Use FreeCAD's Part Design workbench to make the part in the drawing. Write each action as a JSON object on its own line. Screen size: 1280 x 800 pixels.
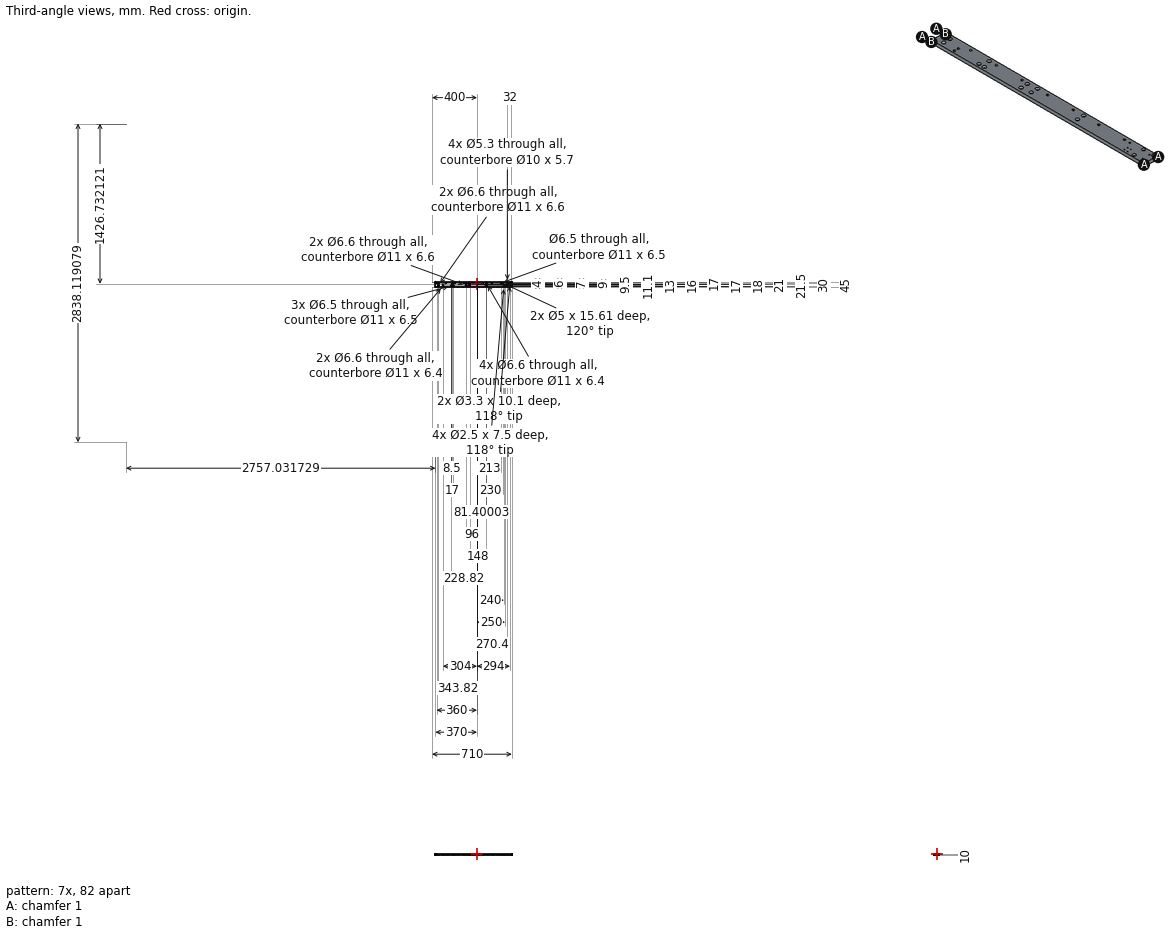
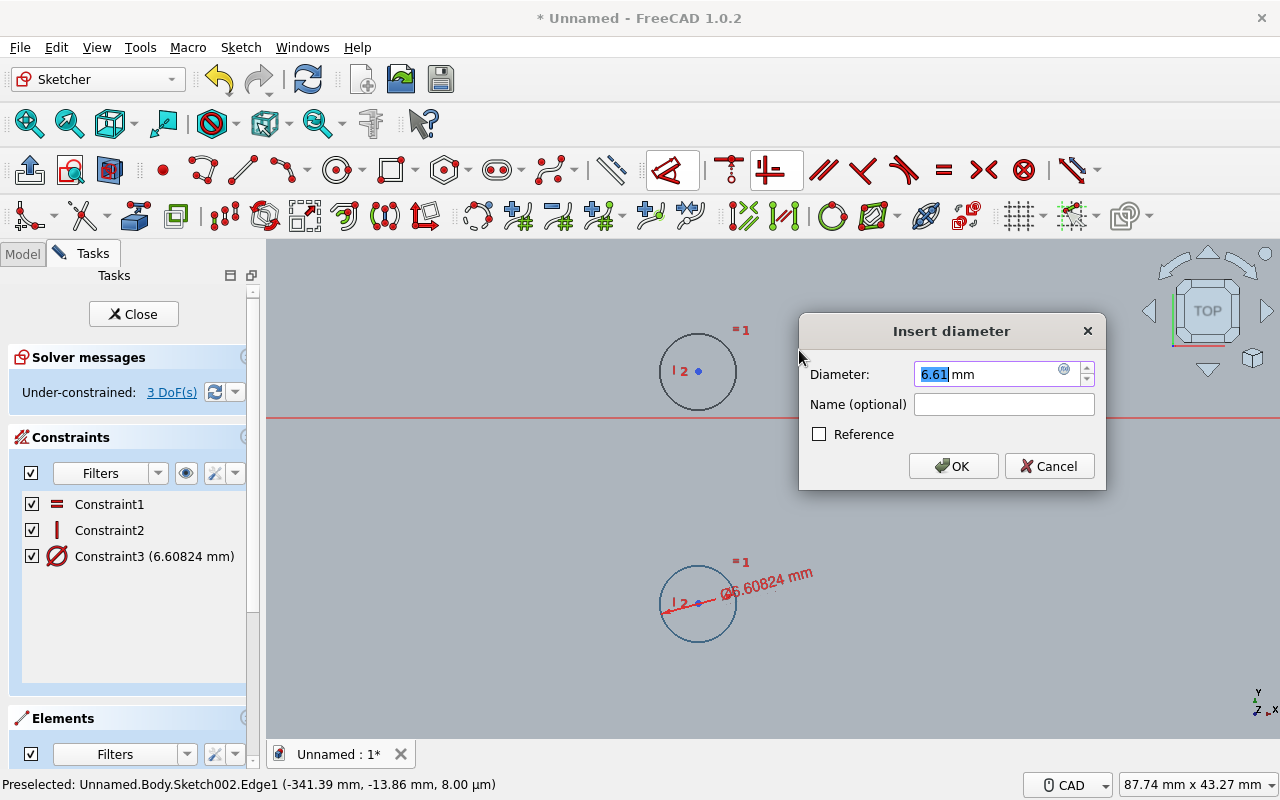
{"action": "type", "text": "6.6"}
{"action": "key", "text": "Return"}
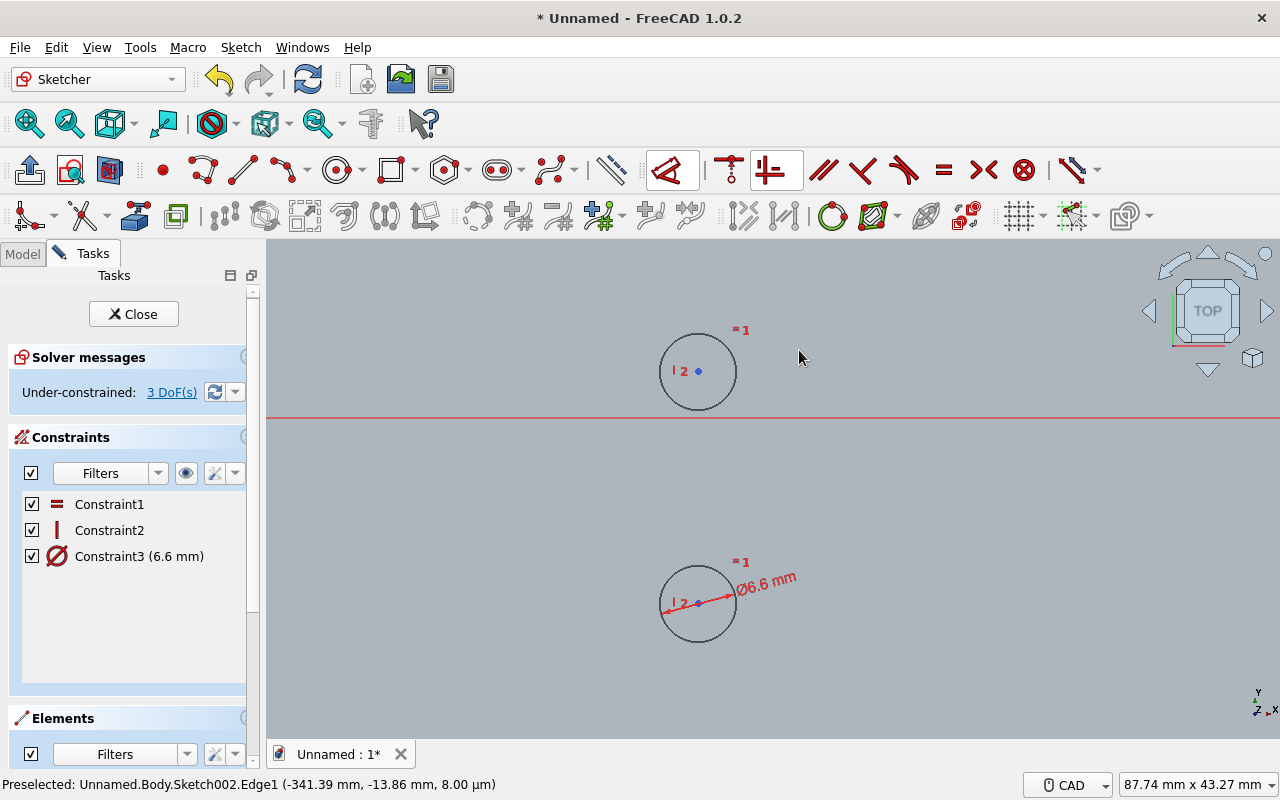
{"action": "left_click", "coordinate": [698, 372]}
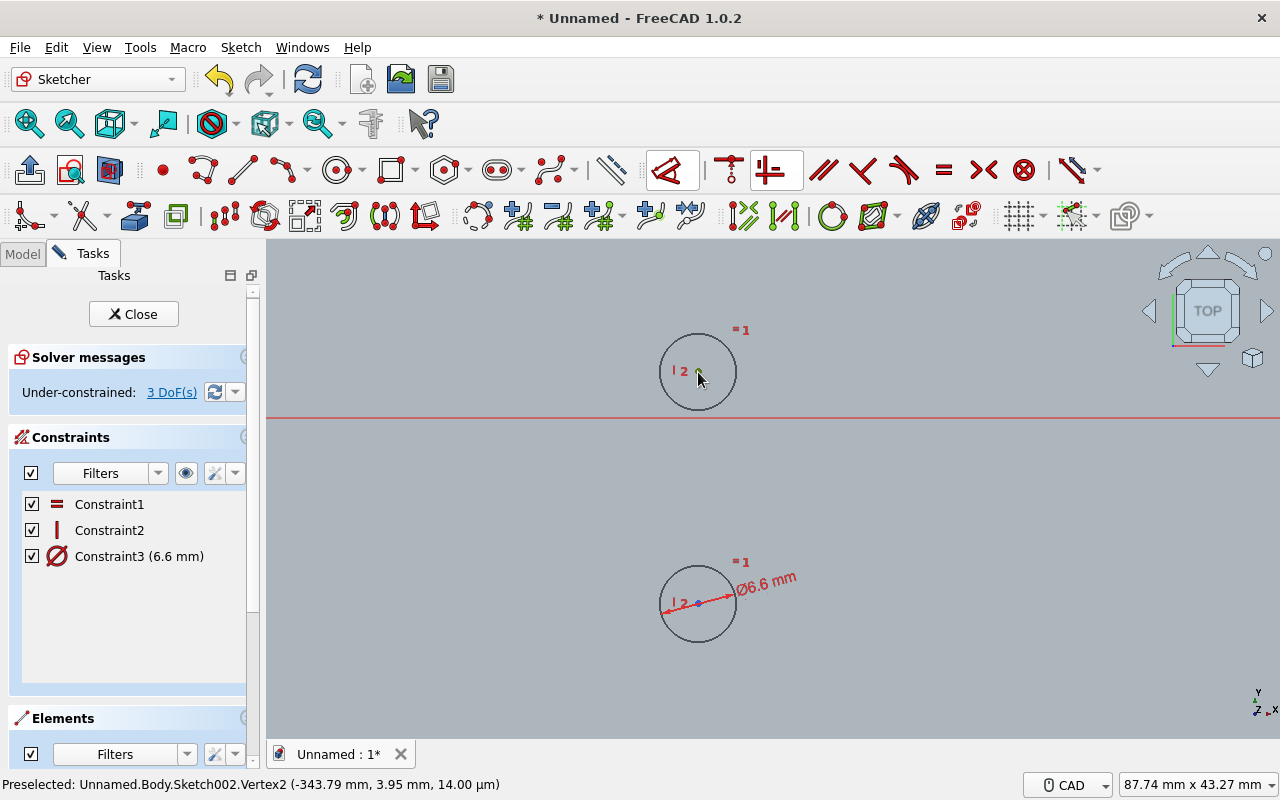
{"action": "left_click", "coordinate": [694, 170]}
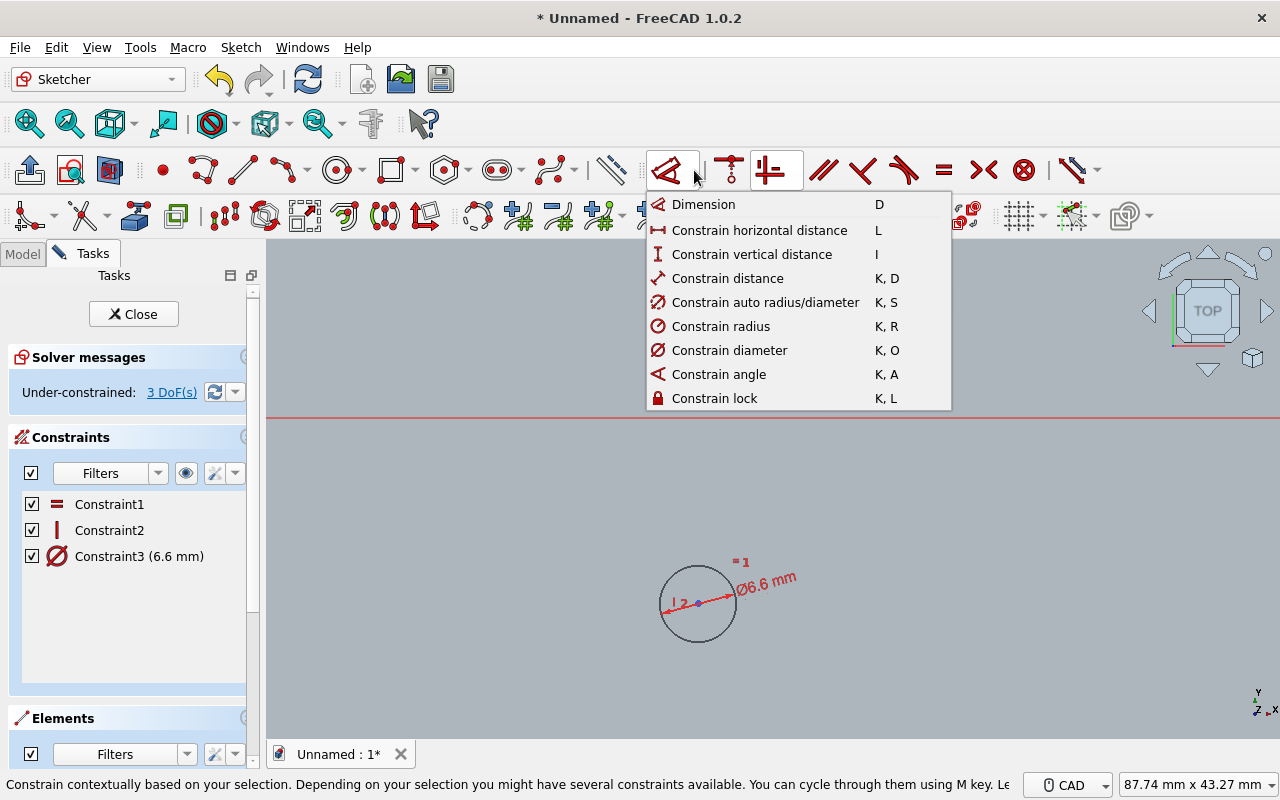
{"action": "left_click", "coordinate": [799, 254]}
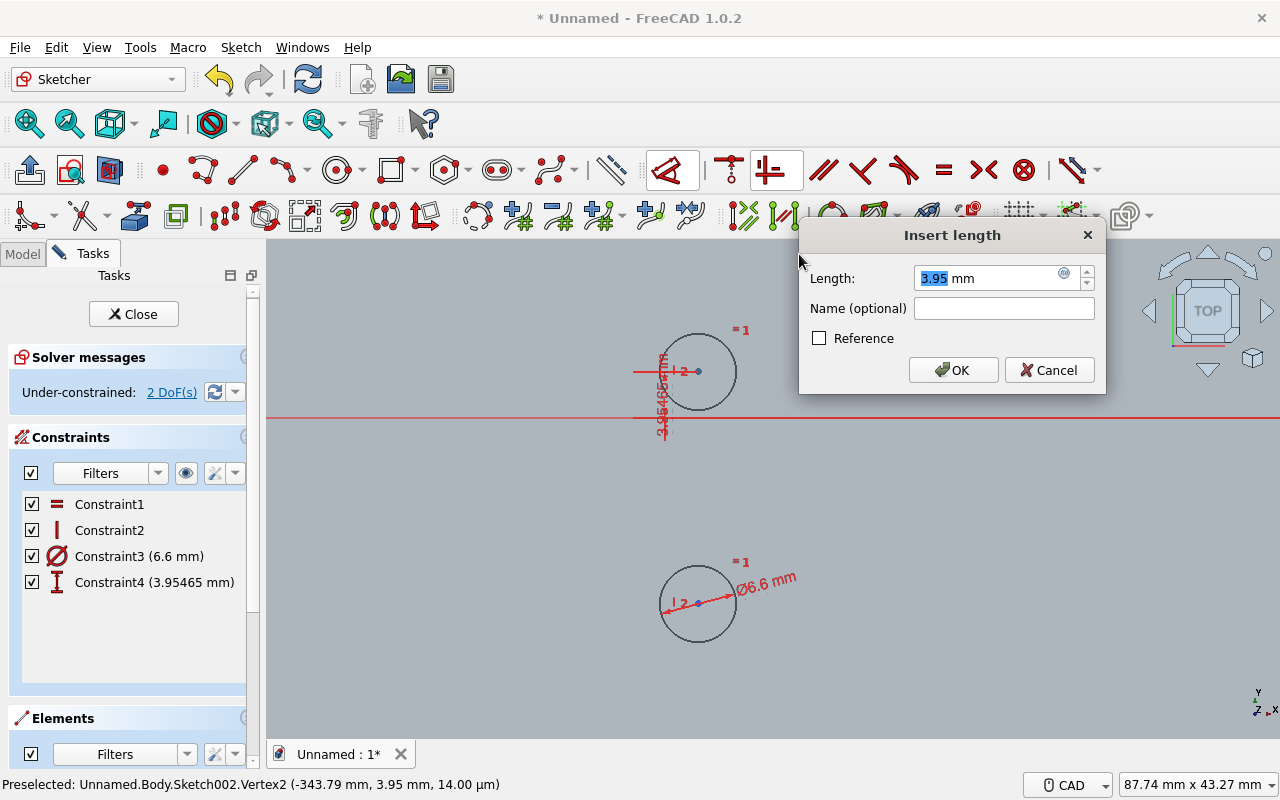
{"action": "type", "text": "4"}
{"action": "key", "text": "Return"}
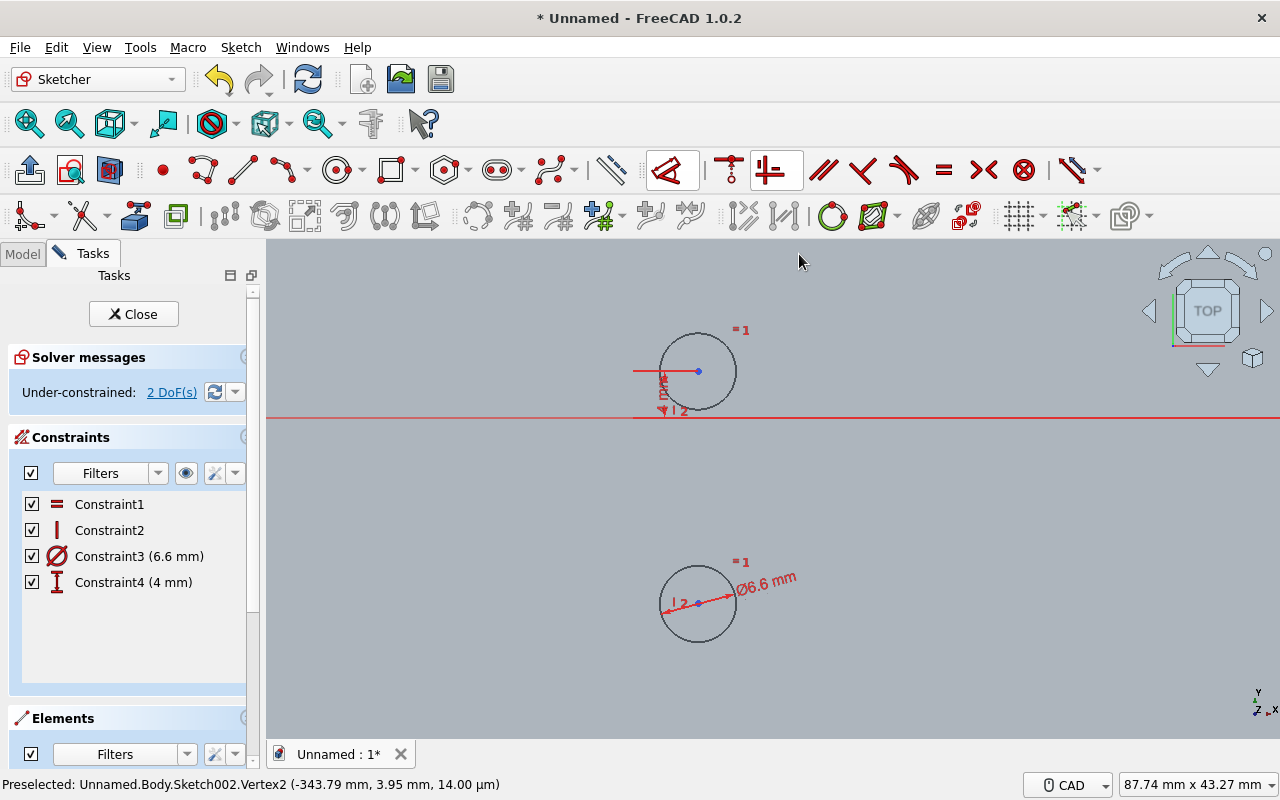
{"action": "left_click", "coordinate": [698, 604]}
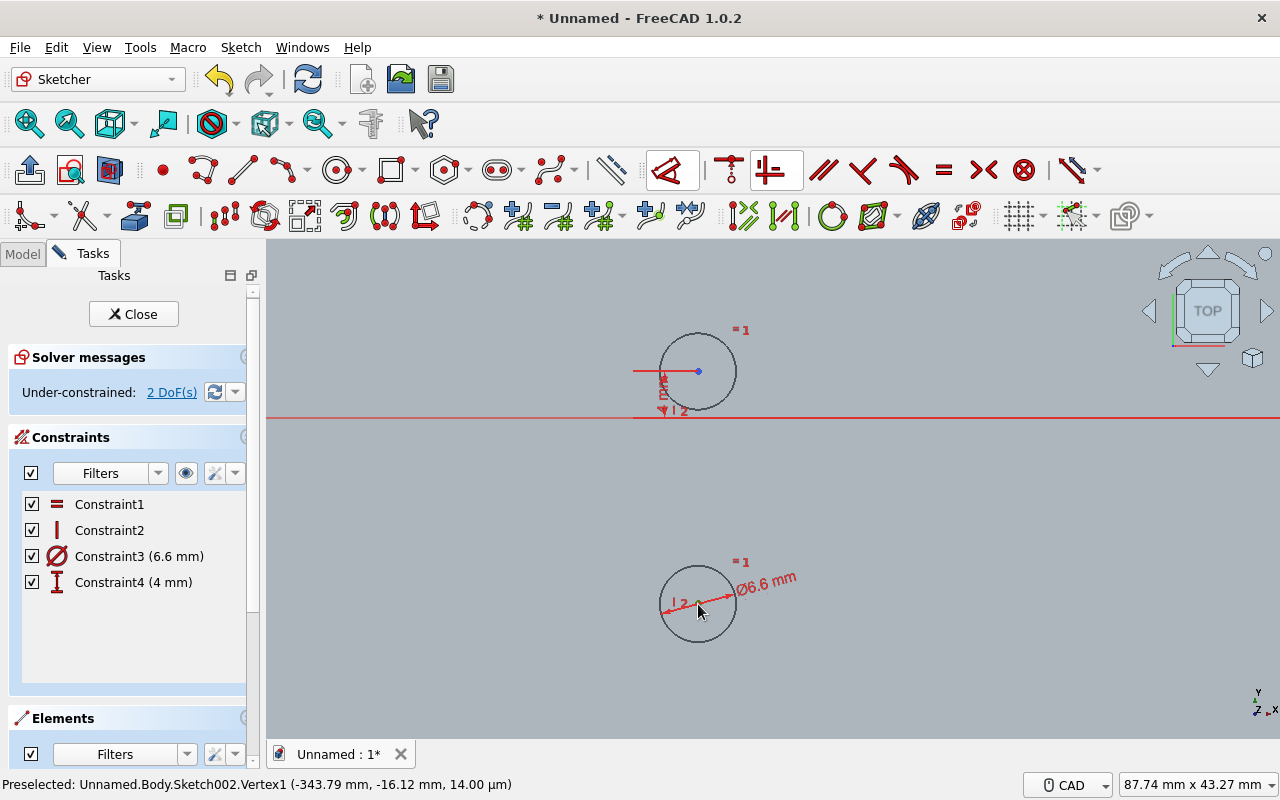
{"action": "key", "text": "i"}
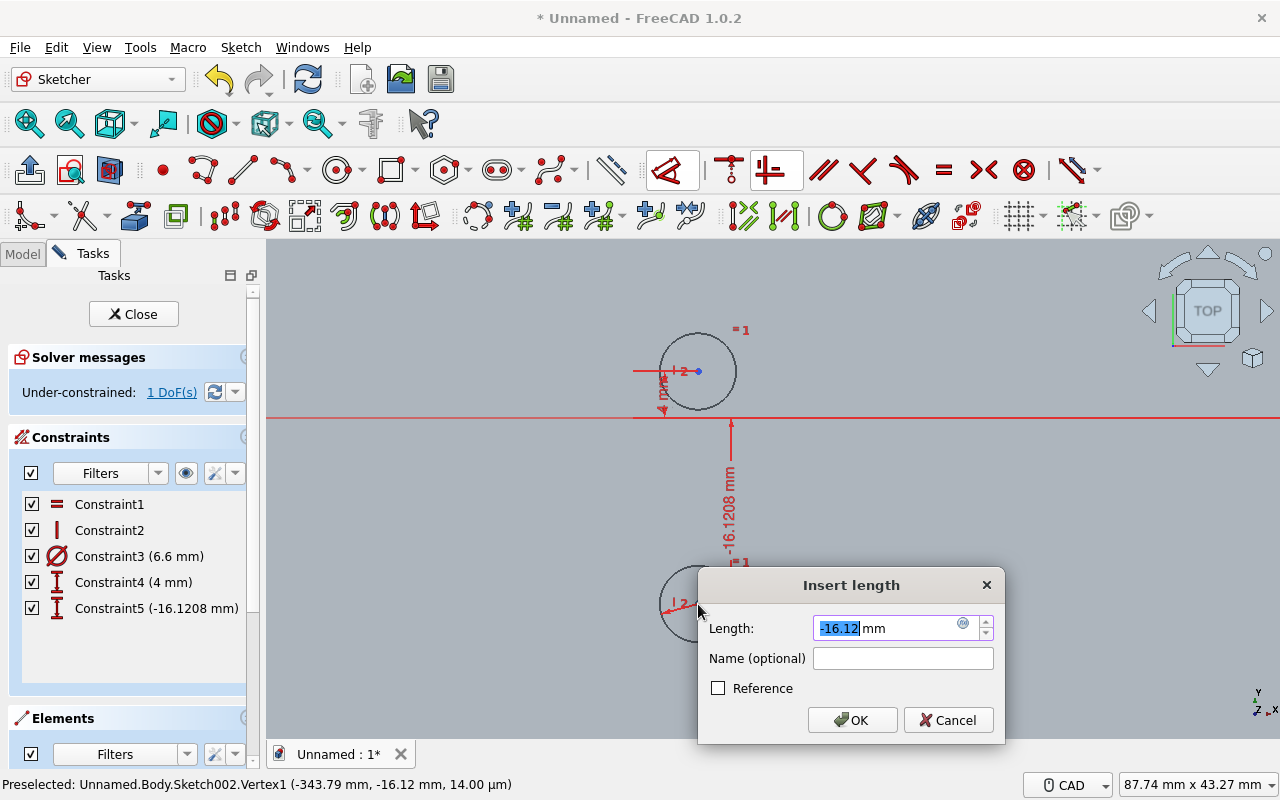
{"action": "type", "text": "-16"}
{"action": "key", "text": "Return"}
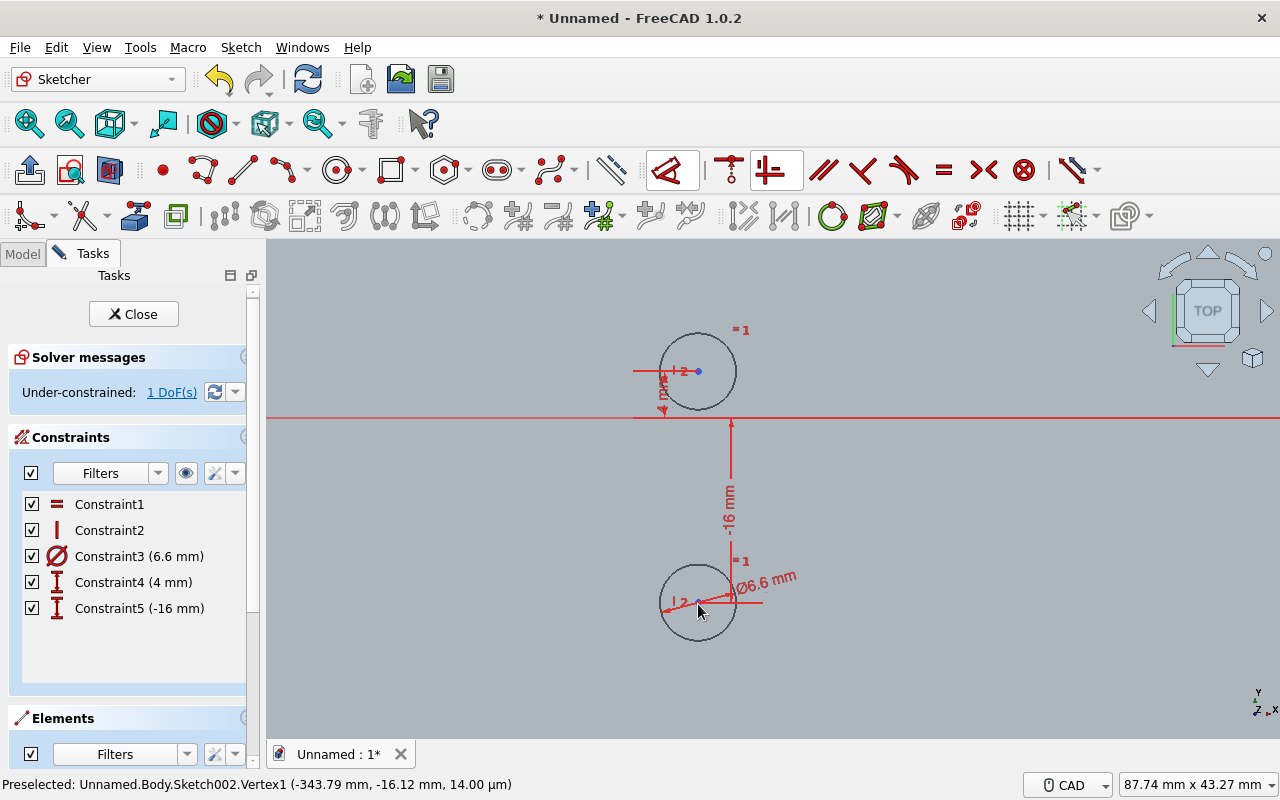
{"action": "left_click", "coordinate": [698, 603]}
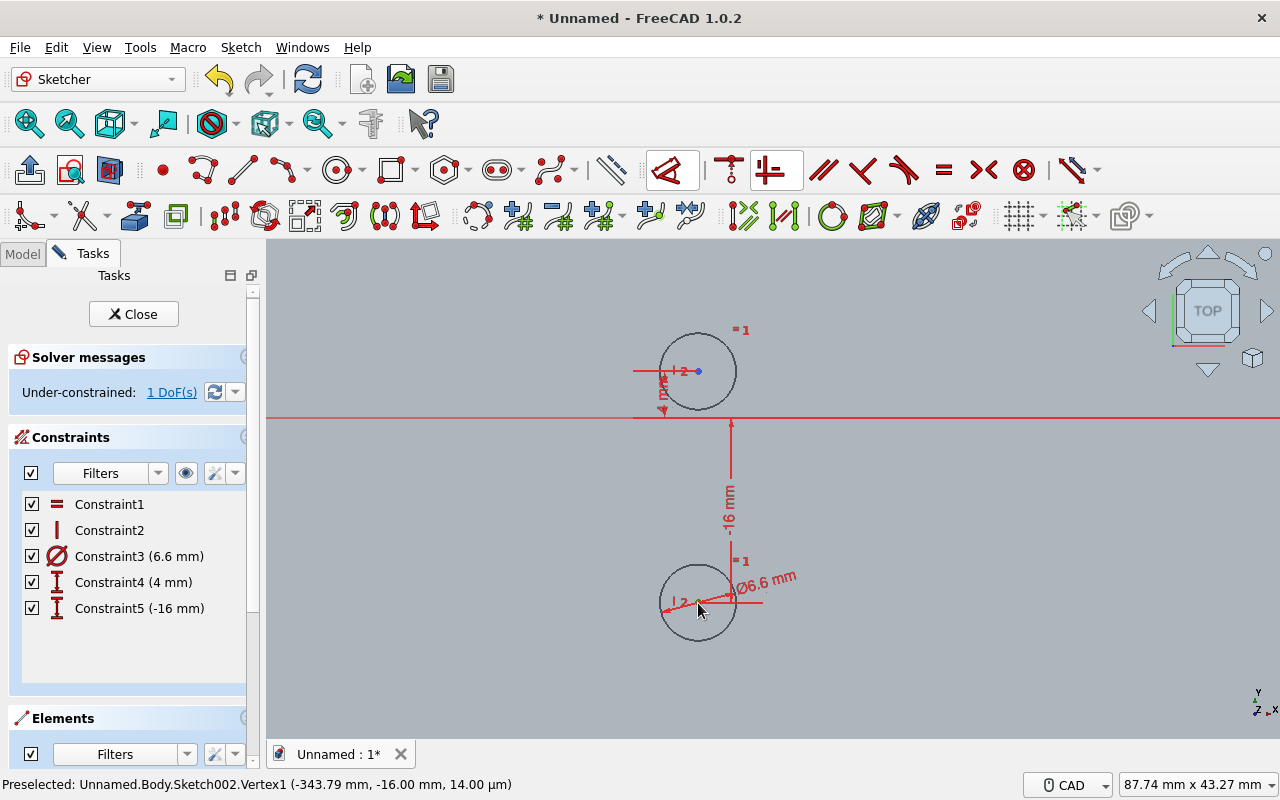
{"action": "key", "text": "l"}